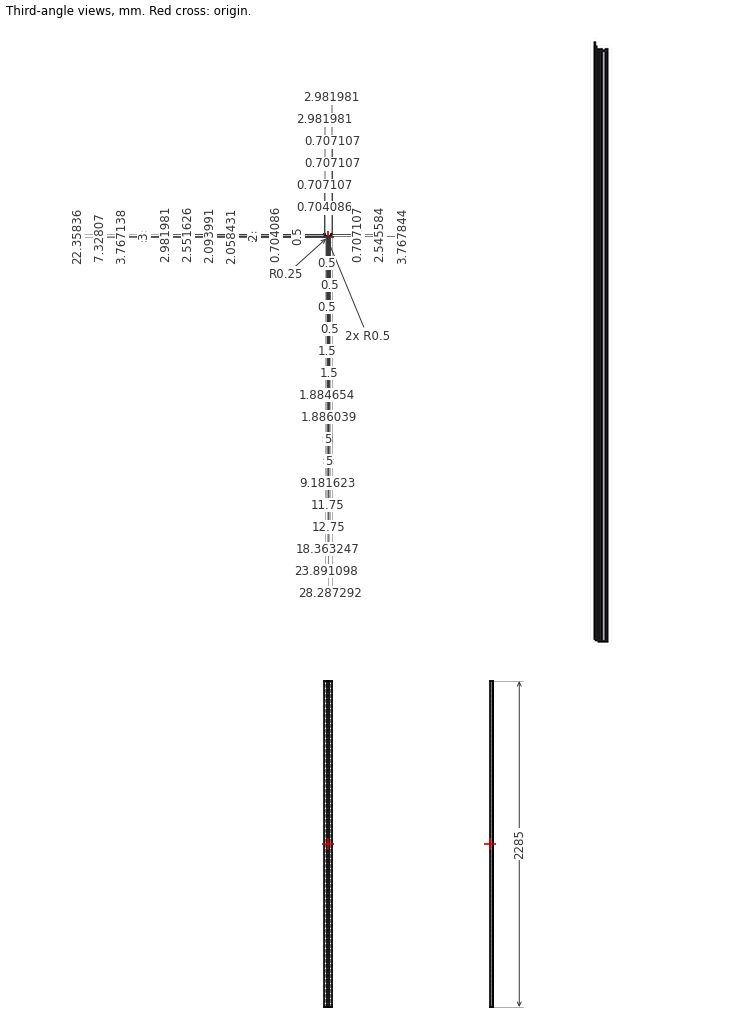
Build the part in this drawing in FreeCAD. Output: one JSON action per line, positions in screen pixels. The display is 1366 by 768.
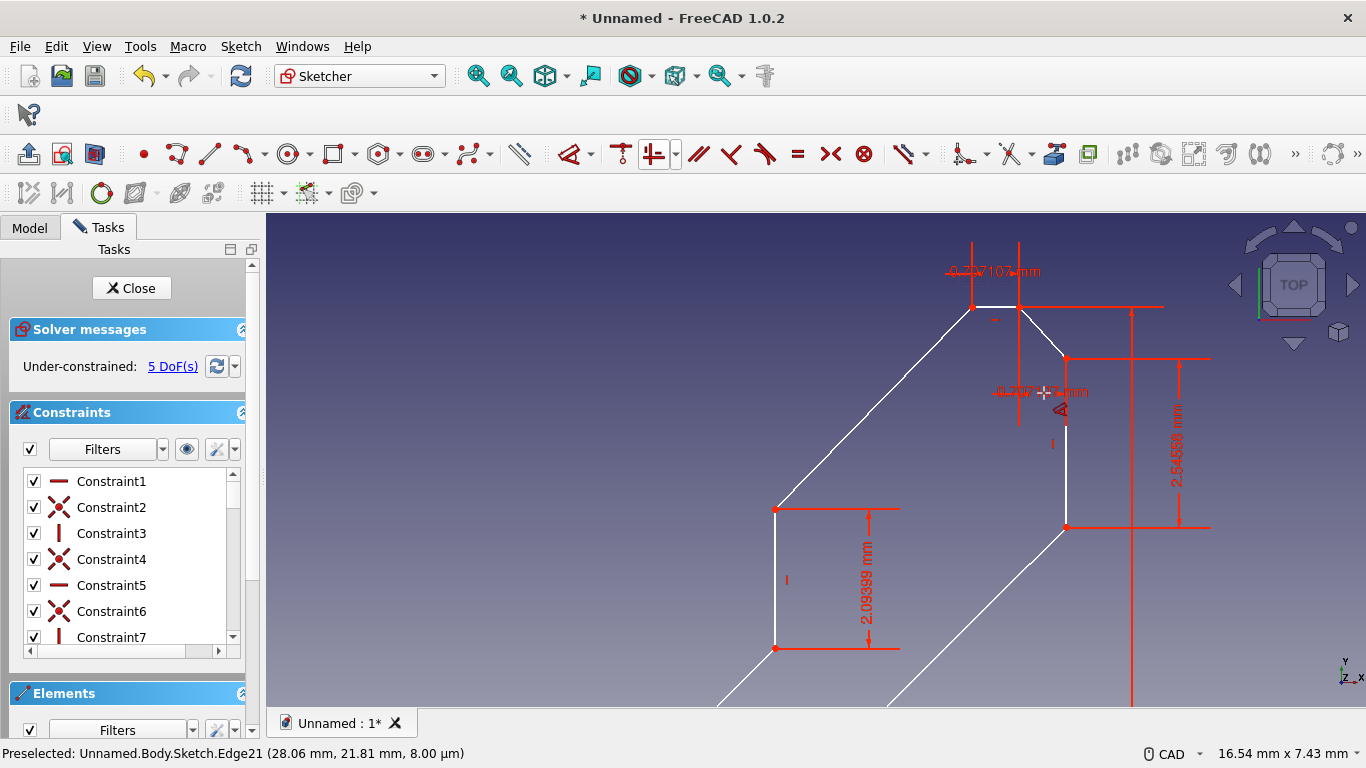
{"action": "left_click", "coordinate": [1052, 343]}
{"action": "left_click", "coordinate": [1100, 333]}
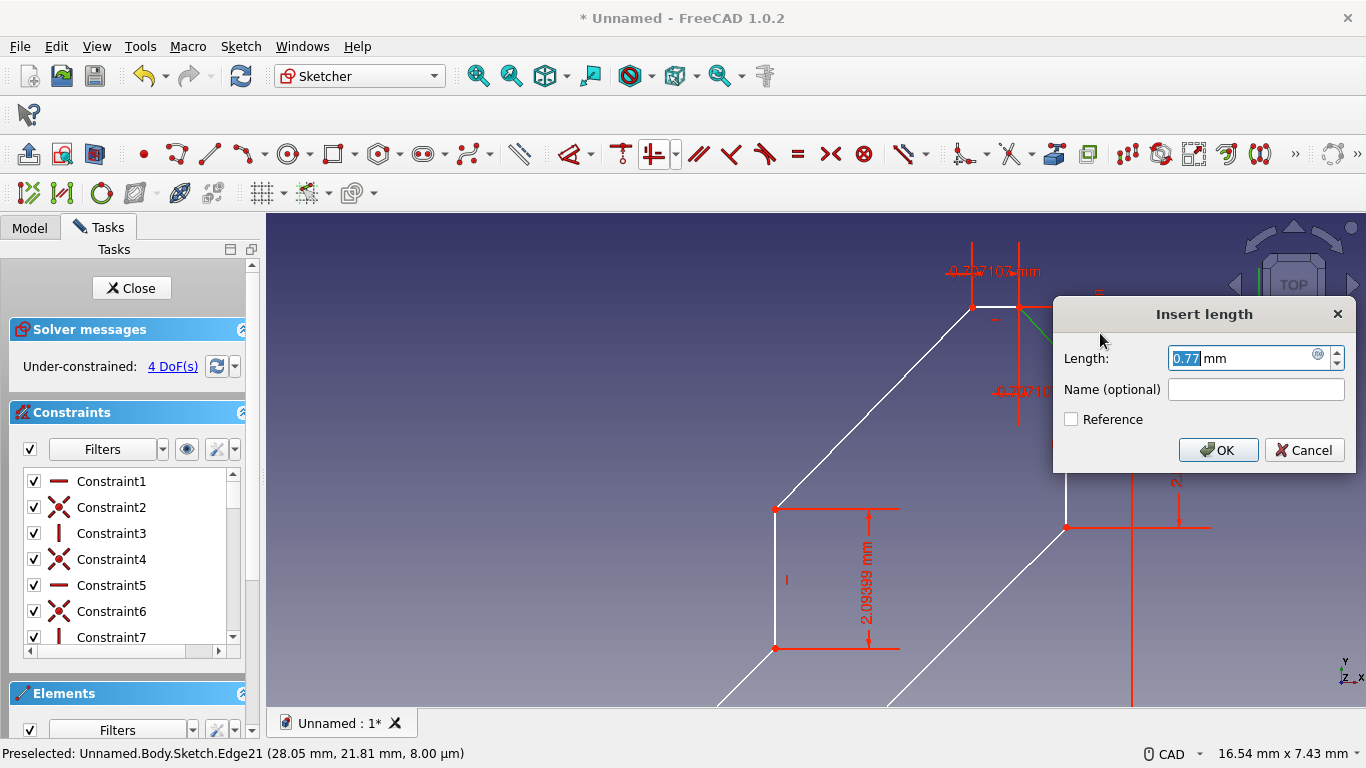
{"action": "type", "text": "0.707107"}
{"action": "key", "text": "Return"}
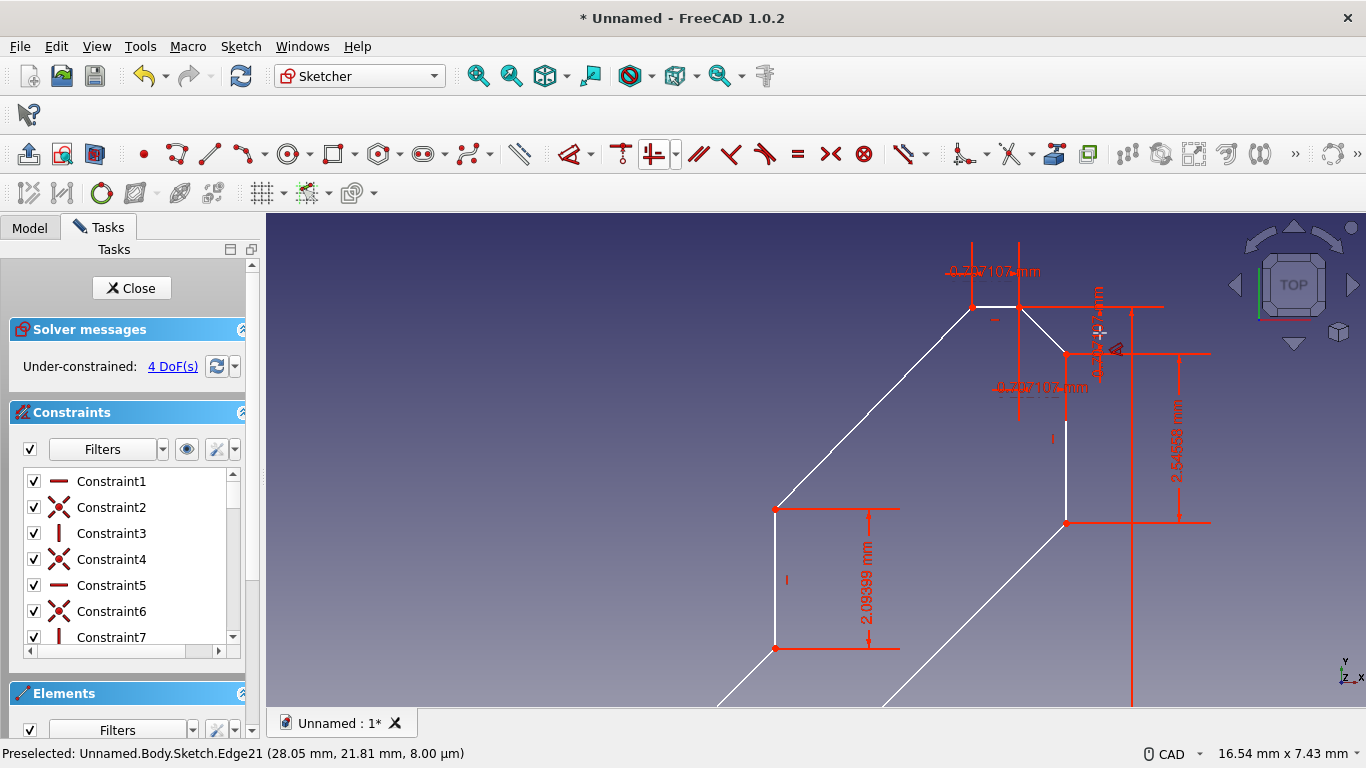
{"action": "scroll", "coordinate": [1057, 343], "scroll_direction": "down", "scroll_amount": 9}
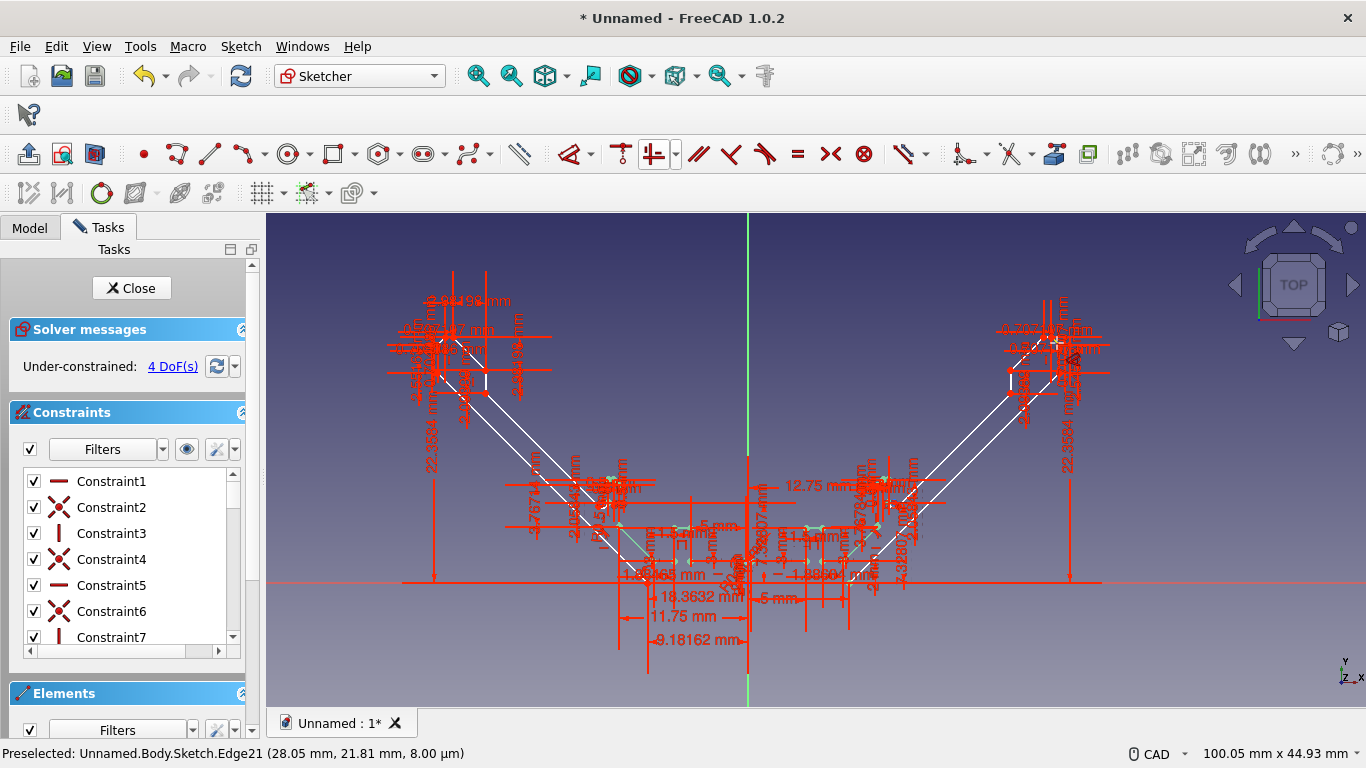
{"action": "left_click", "coordinate": [1034, 347]}
{"action": "left_click", "coordinate": [1027, 303]}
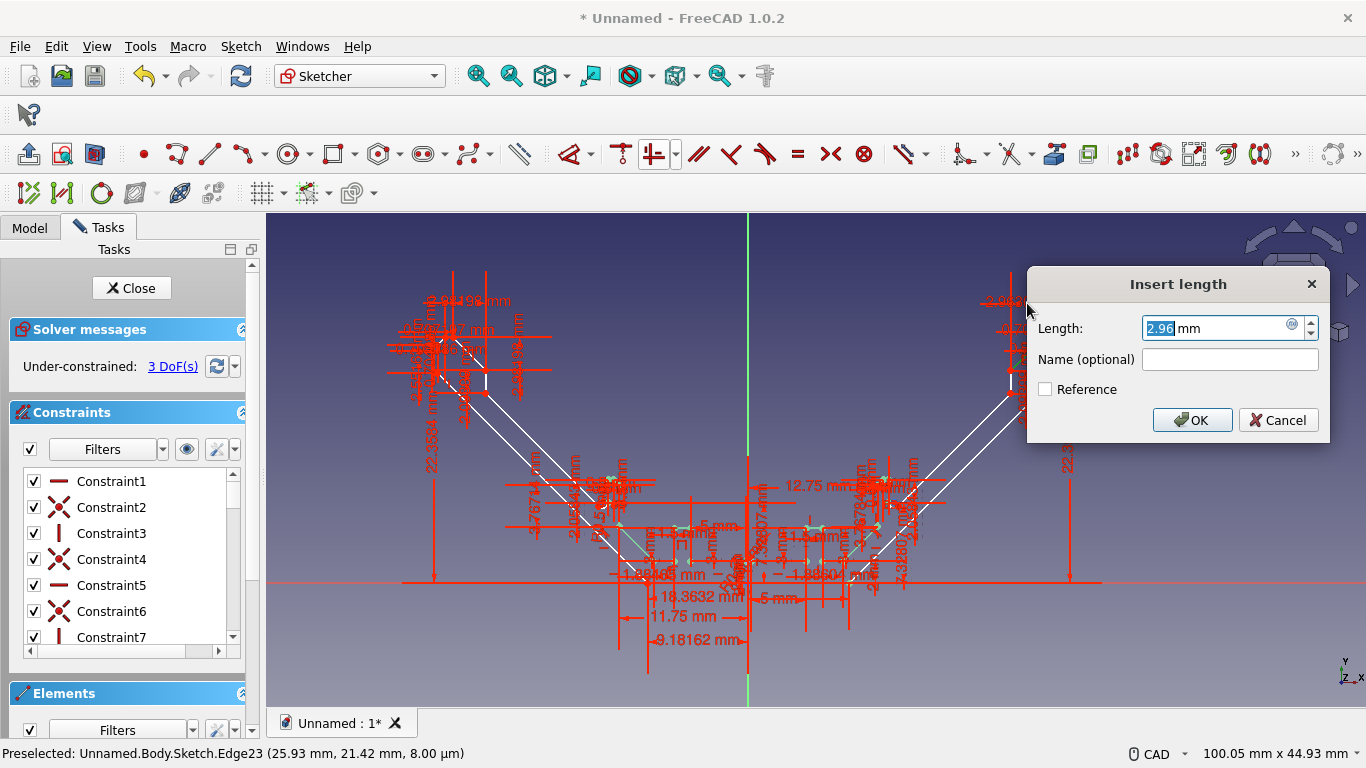
{"action": "type", "text": "2.981981"}
{"action": "key", "text": "Return"}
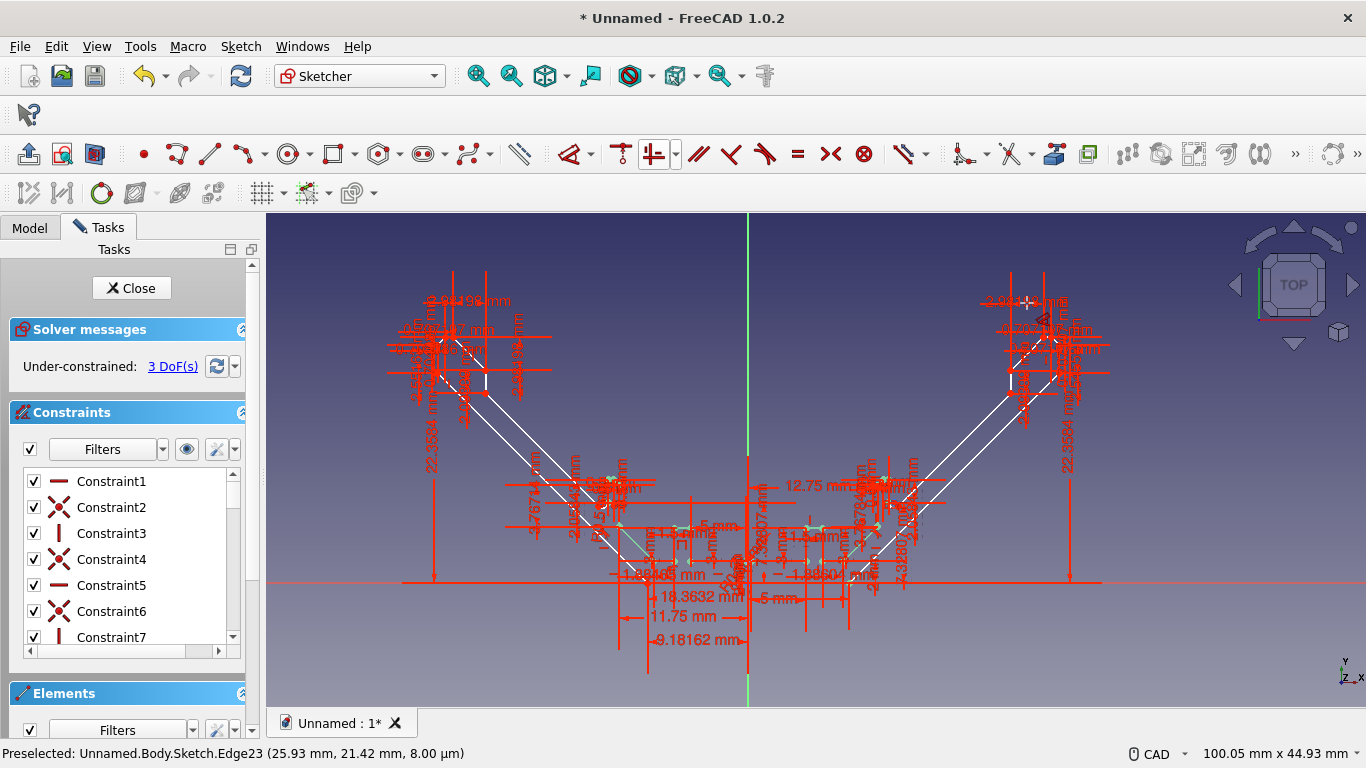
{"action": "left_click", "coordinate": [1034, 347]}
{"action": "left_click", "coordinate": [977, 354]}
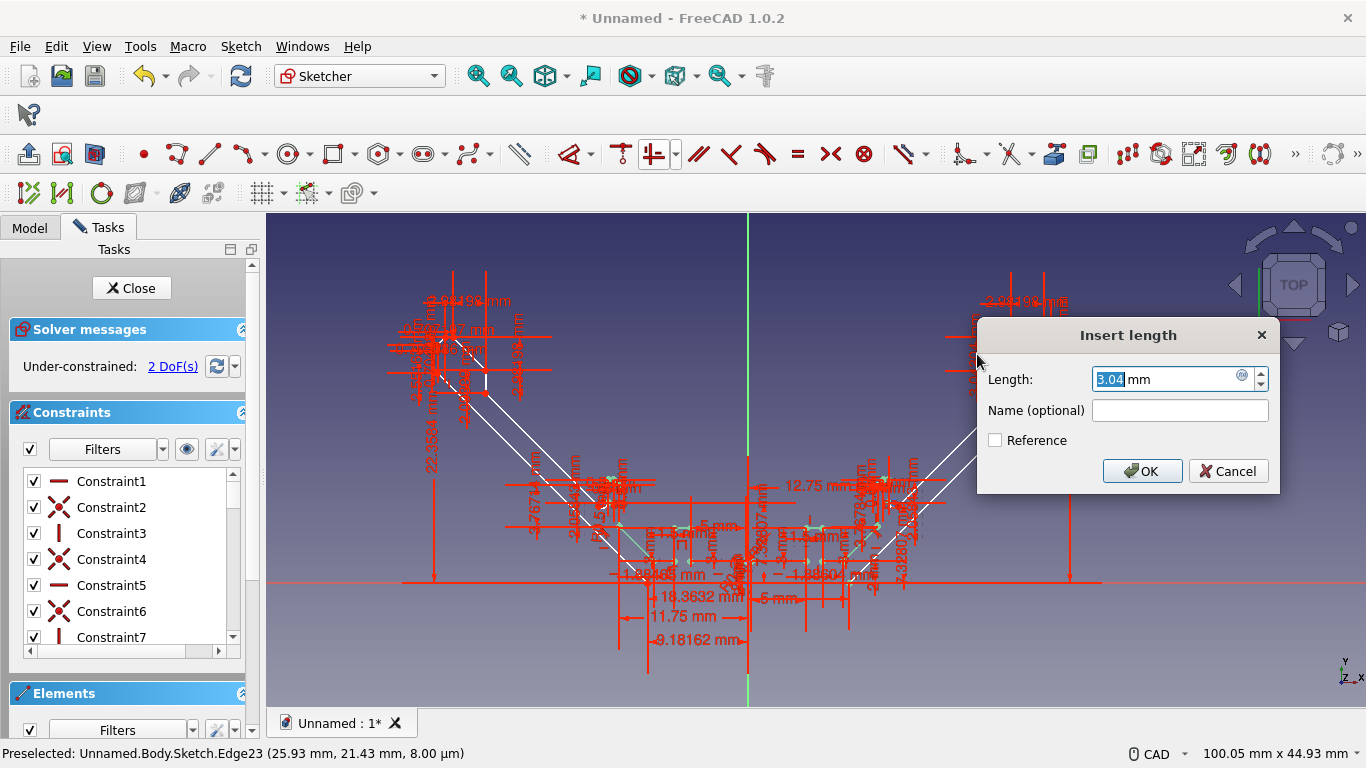
{"action": "type", "text": "2.981981"}
{"action": "key", "text": "Return"}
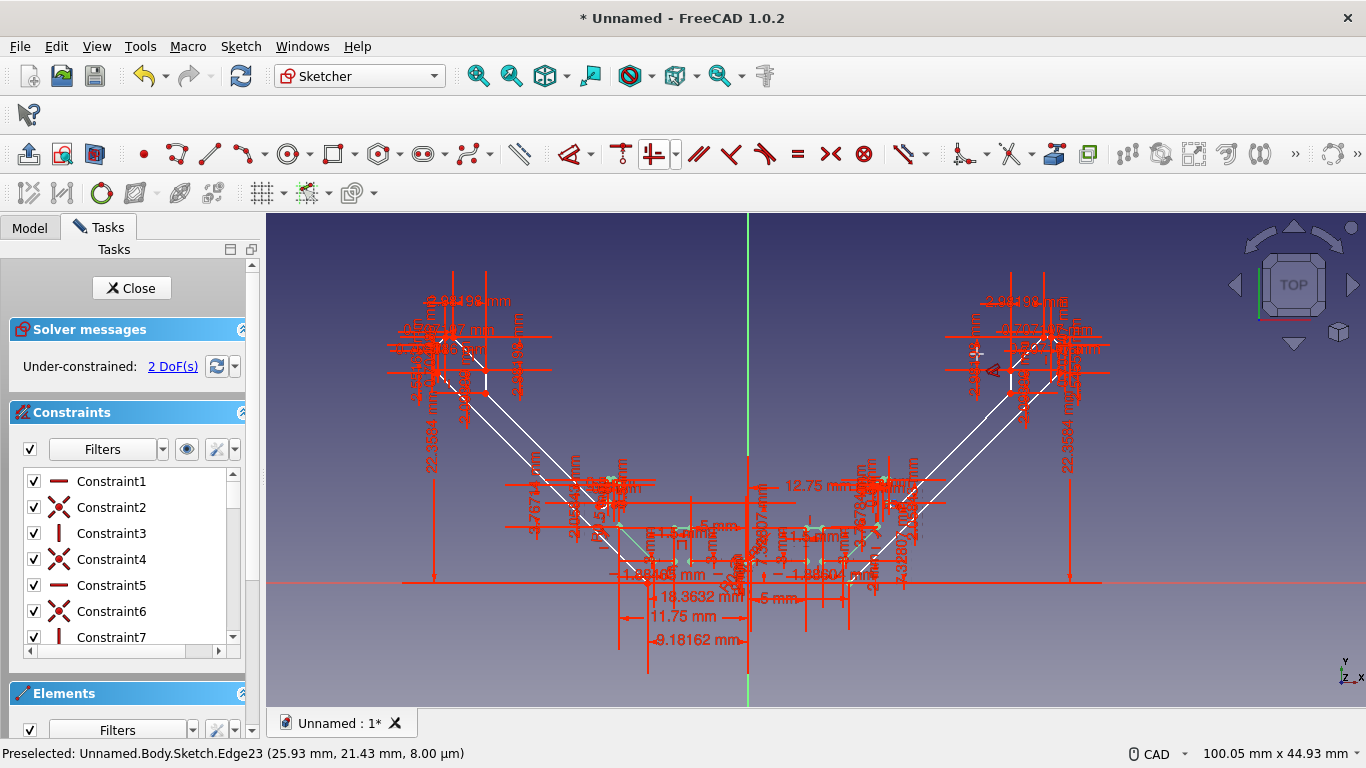
{"action": "left_click", "coordinate": [486, 393]}
{"action": "left_click", "coordinate": [557, 617]}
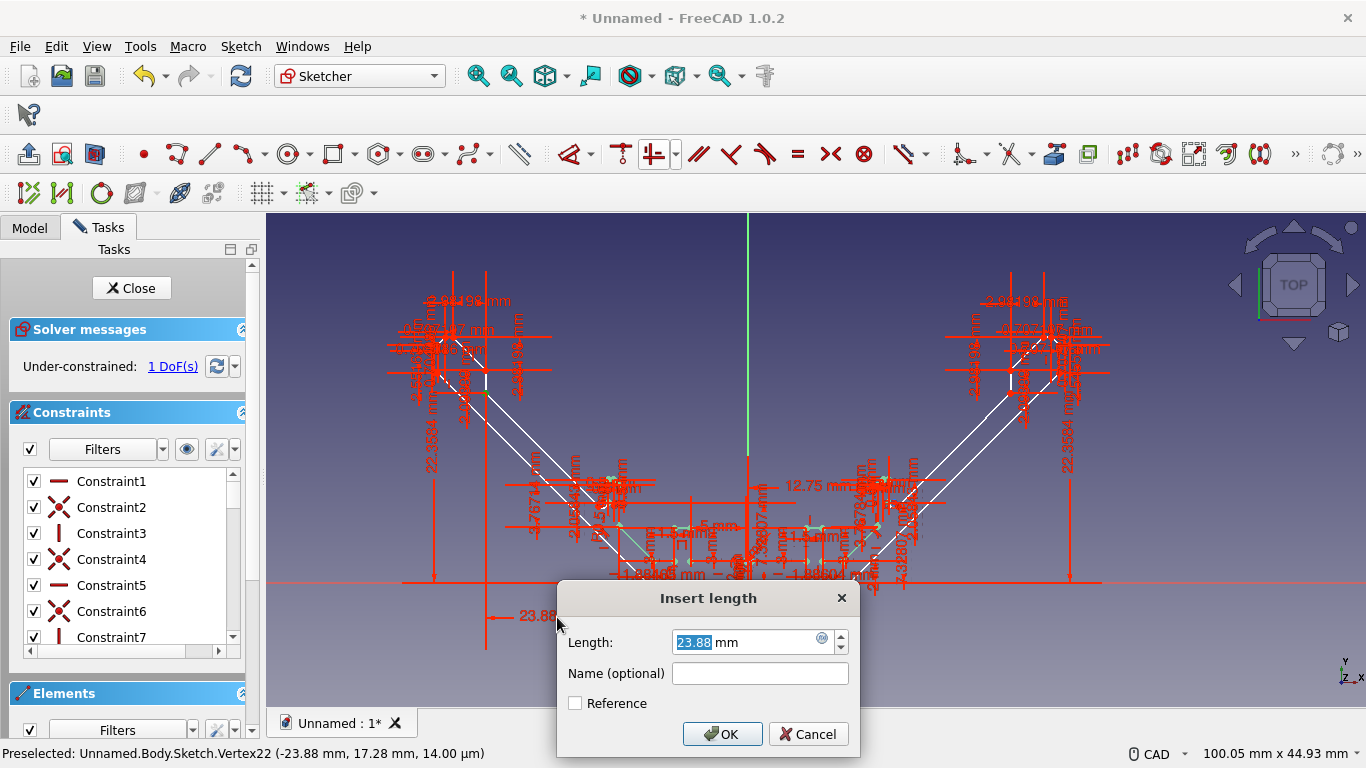
{"action": "type", "text": "23.891098"}
{"action": "key", "text": "Return"}